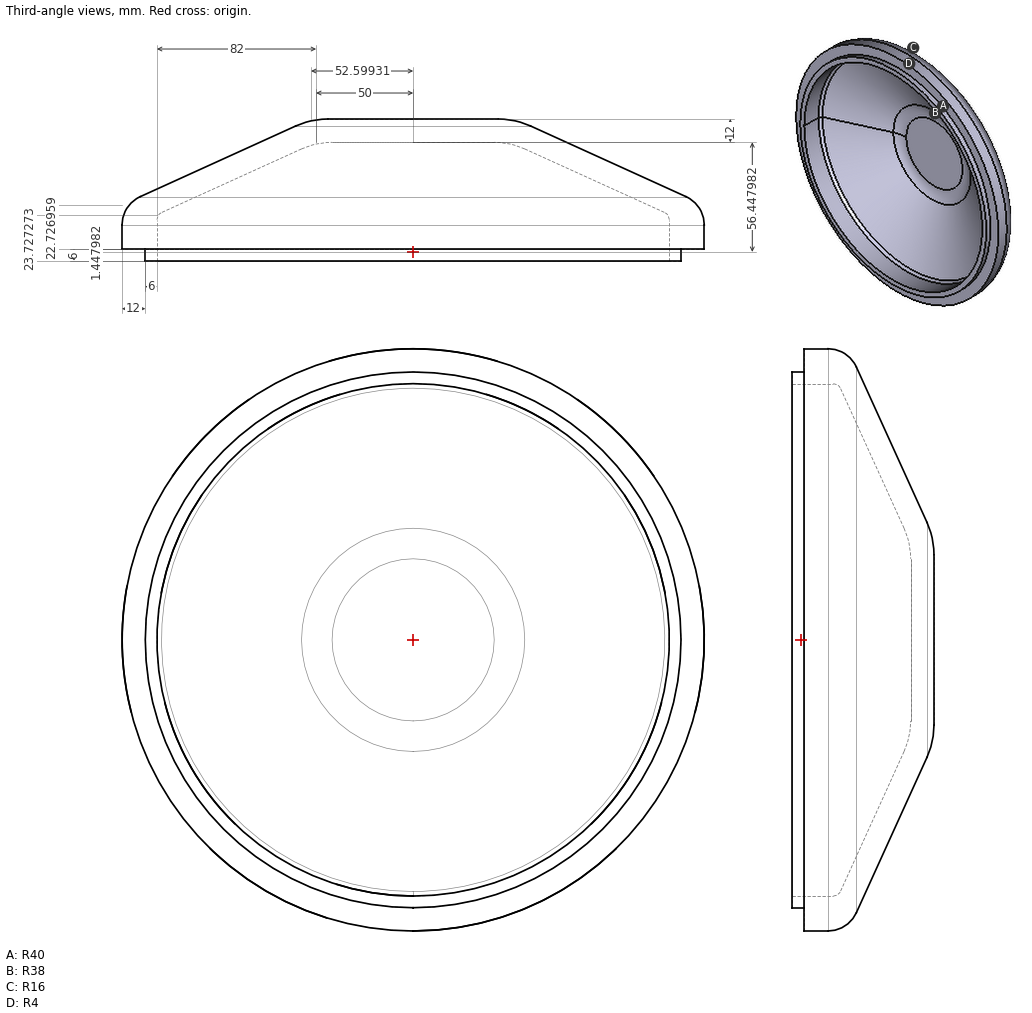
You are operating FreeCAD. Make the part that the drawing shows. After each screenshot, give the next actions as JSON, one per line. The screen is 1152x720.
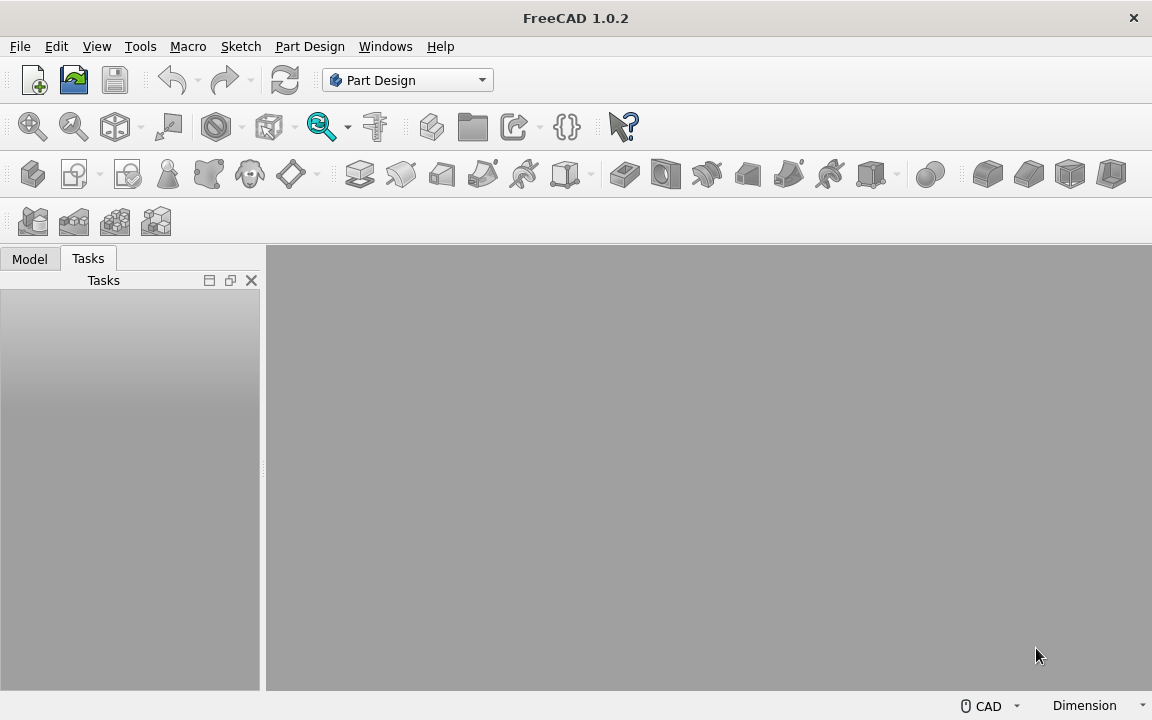
{"action": "key", "text": "ctrl+n"}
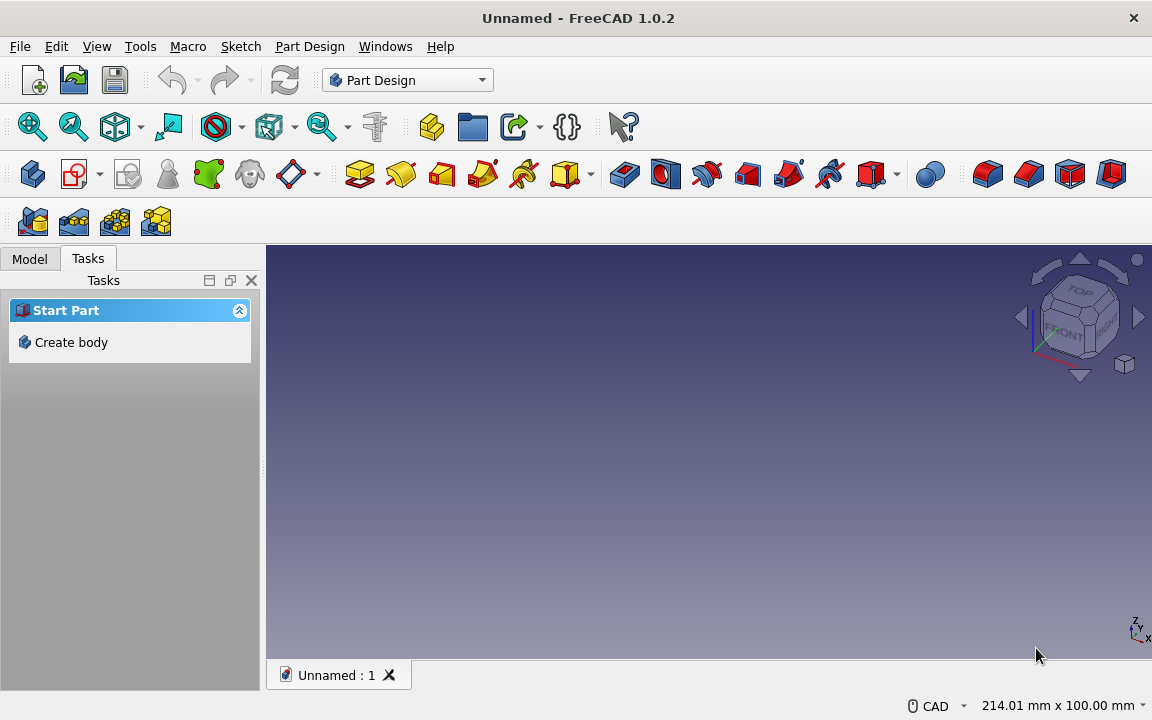
{"action": "left_click", "coordinate": [74, 174]}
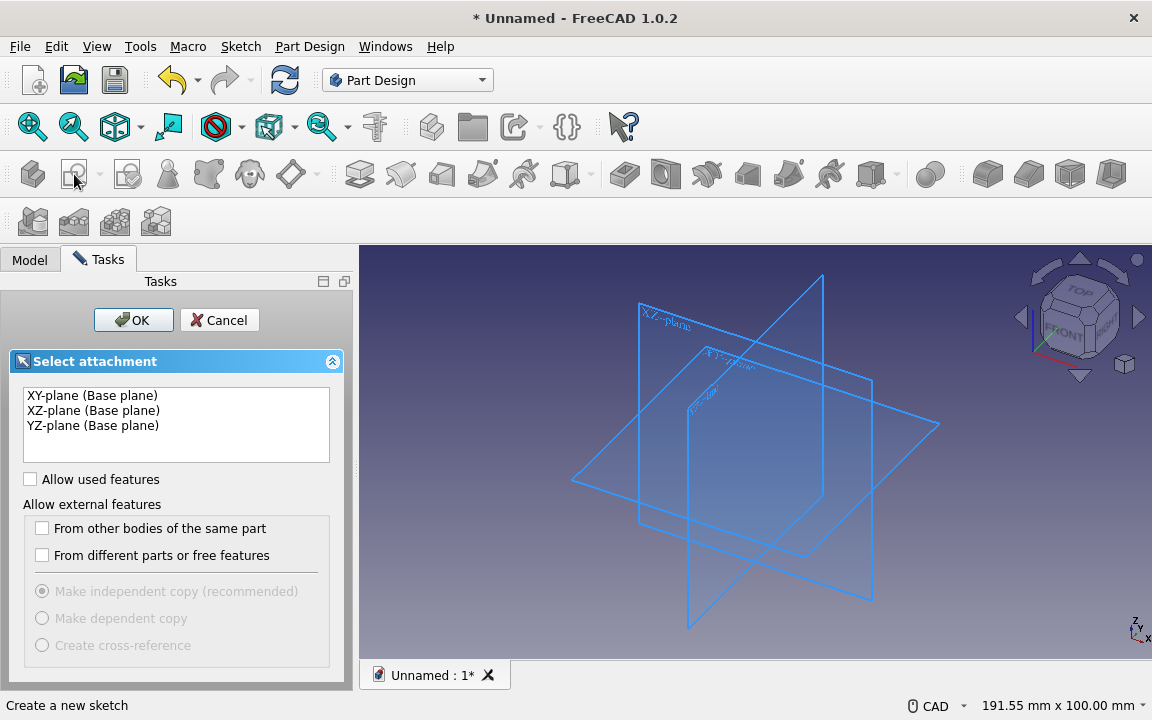
{"action": "left_click", "coordinate": [84, 396]}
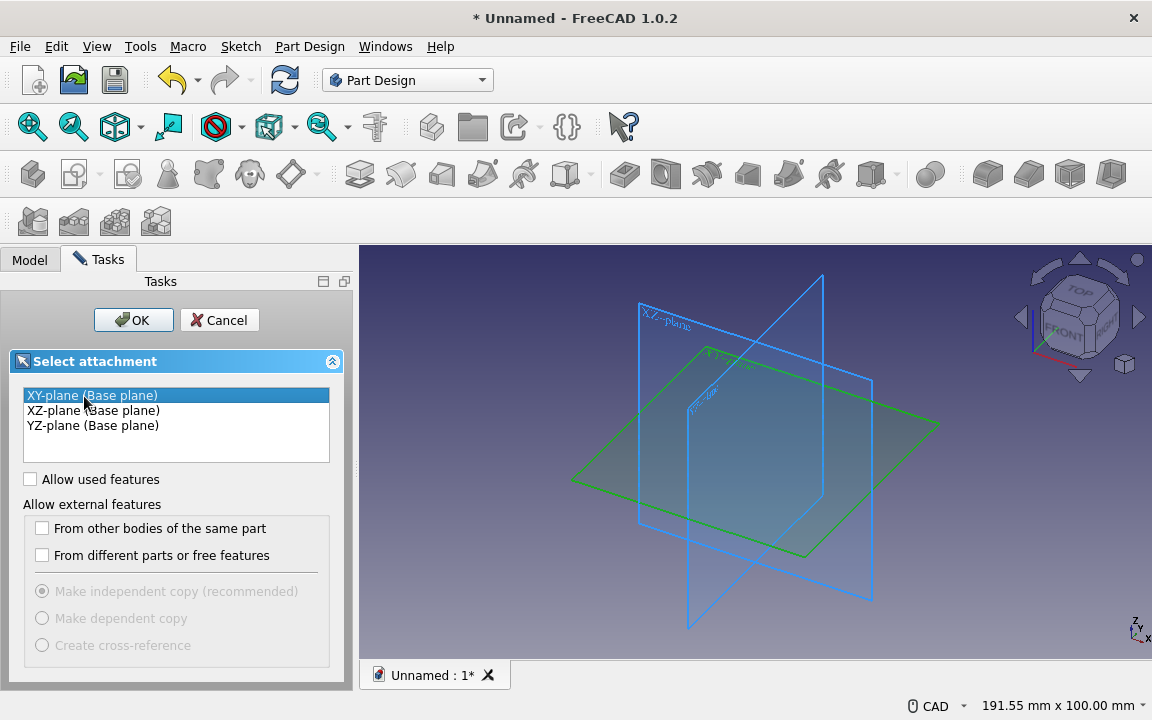
{"action": "left_click", "coordinate": [134, 320]}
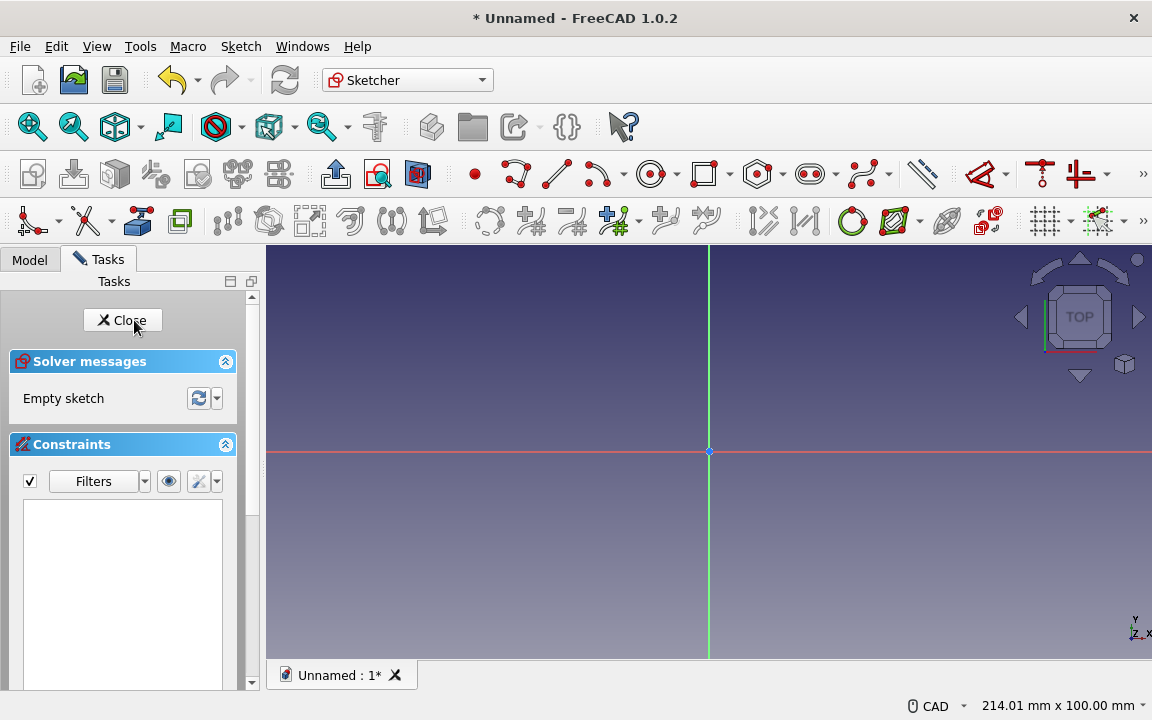
{"action": "scroll", "coordinate": [987, 631], "scroll_direction": "down", "scroll_amount": 2}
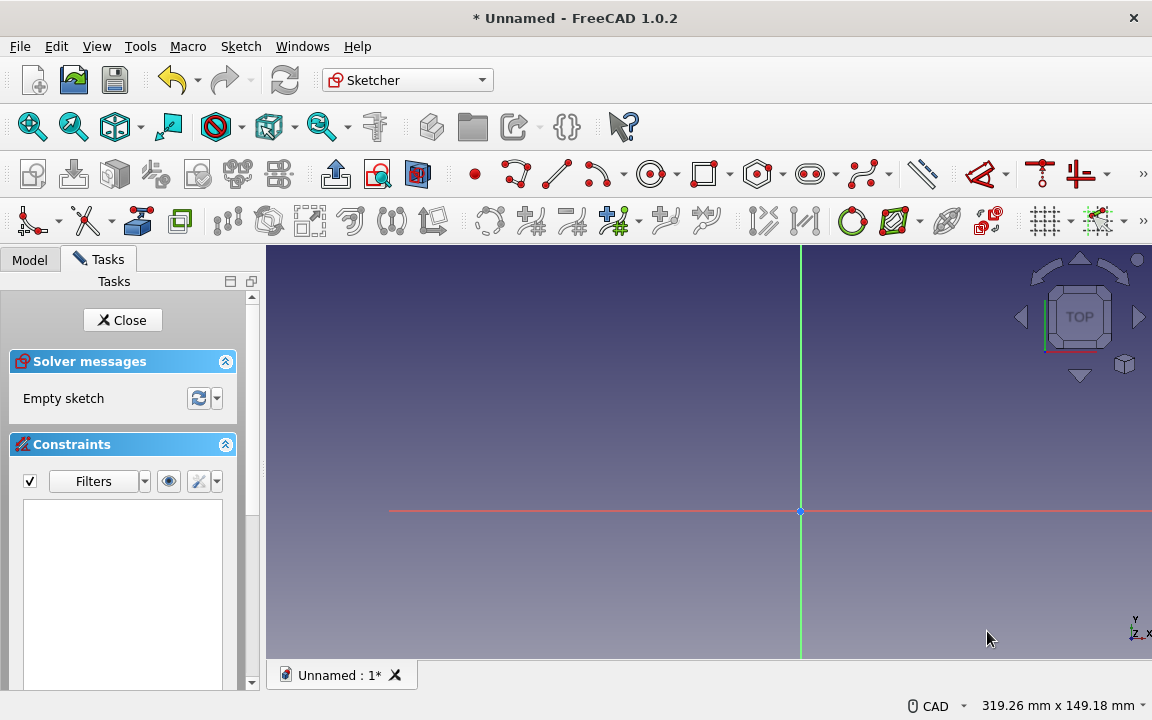
{"action": "key", "text": "g m"}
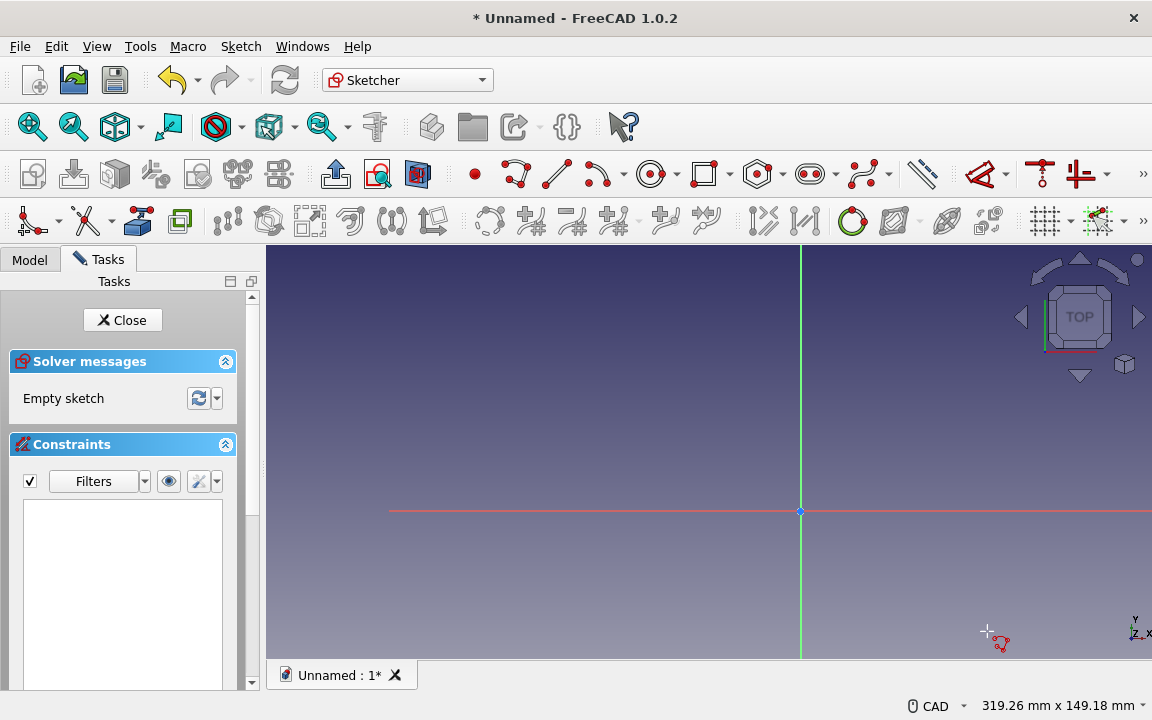
{"action": "left_click", "coordinate": [801, 355]}
{"action": "left_click", "coordinate": [792, 321]}
{"action": "left_click", "coordinate": [655, 321]}
{"action": "left_click", "coordinate": [385, 444]}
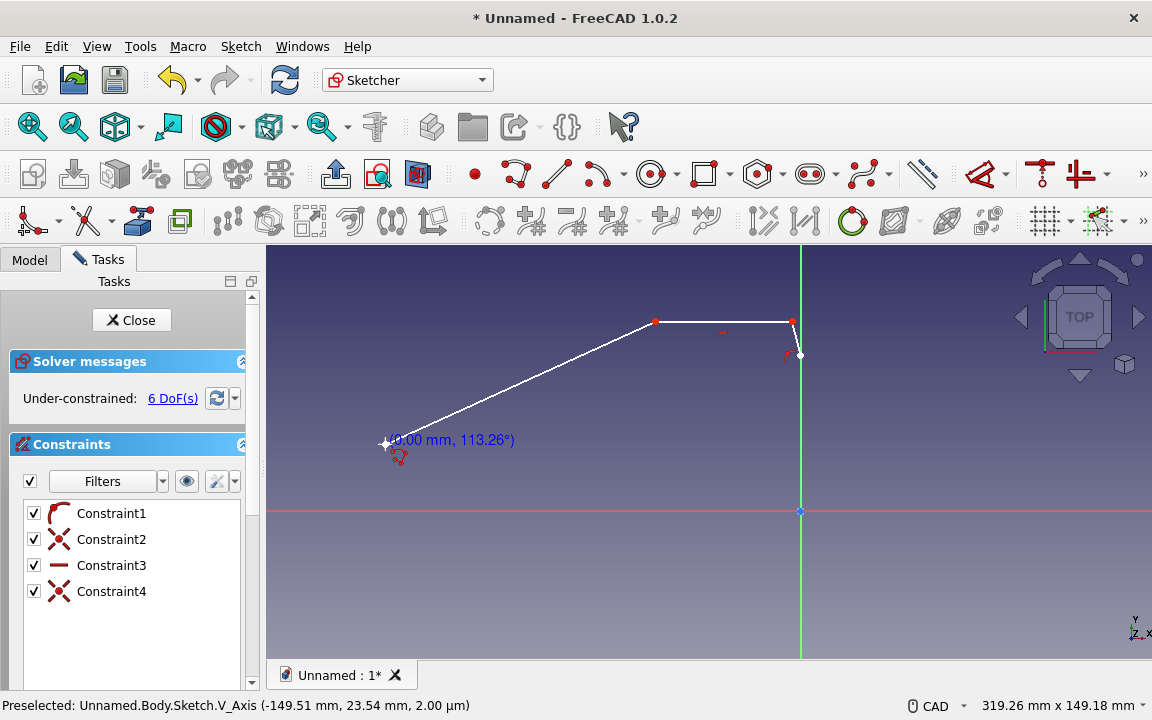
{"action": "scroll", "coordinate": [385, 507], "scroll_direction": "up", "scroll_amount": 7}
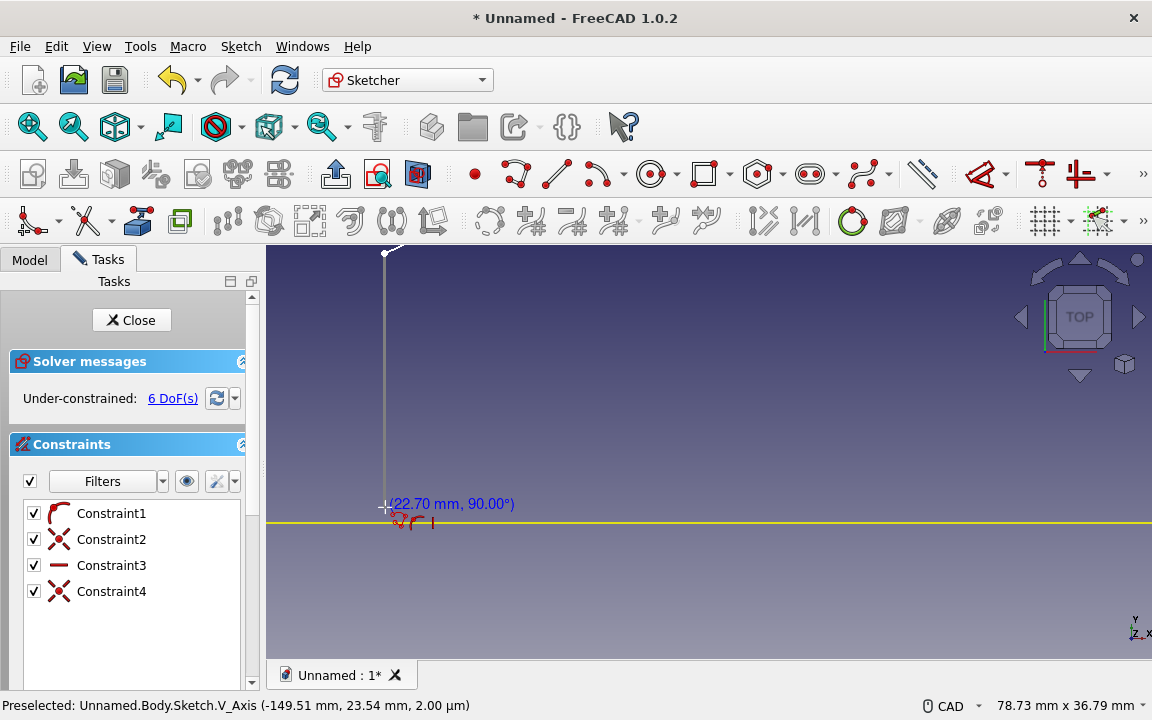
{"action": "left_click", "coordinate": [385, 506]}
{"action": "left_click", "coordinate": [518, 506]}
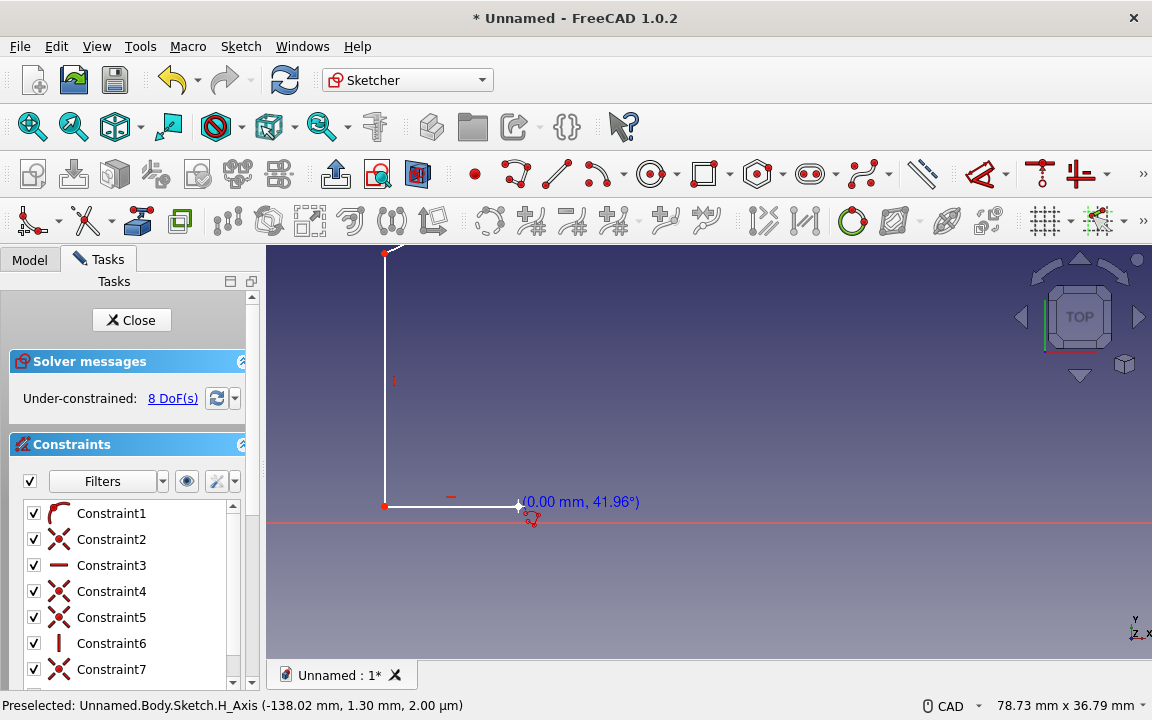
{"action": "scroll", "coordinate": [388, 577], "scroll_direction": "down", "scroll_amount": 6}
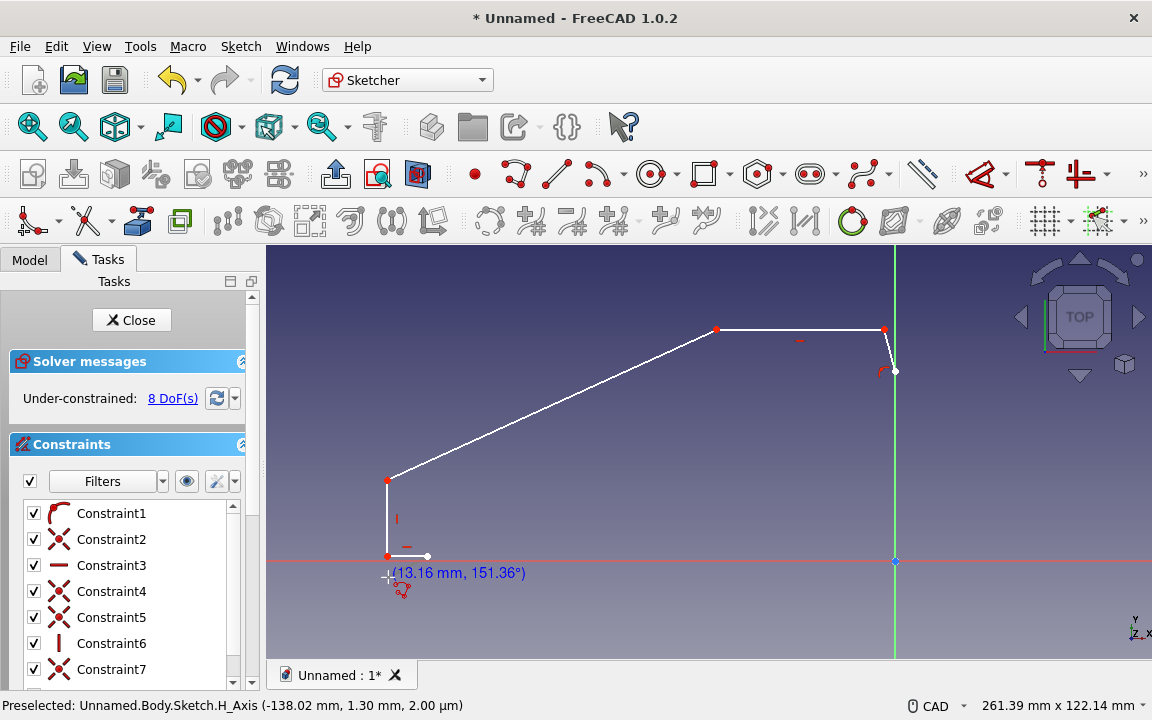
{"action": "left_click", "coordinate": [427, 577]}
{"action": "left_click", "coordinate": [448, 577]}
{"action": "left_click", "coordinate": [448, 496]}
{"action": "left_click", "coordinate": [726, 370]}
{"action": "left_click", "coordinate": [895, 371]}
{"action": "key", "text": "Escape"}
{"action": "key", "text": "Escape"}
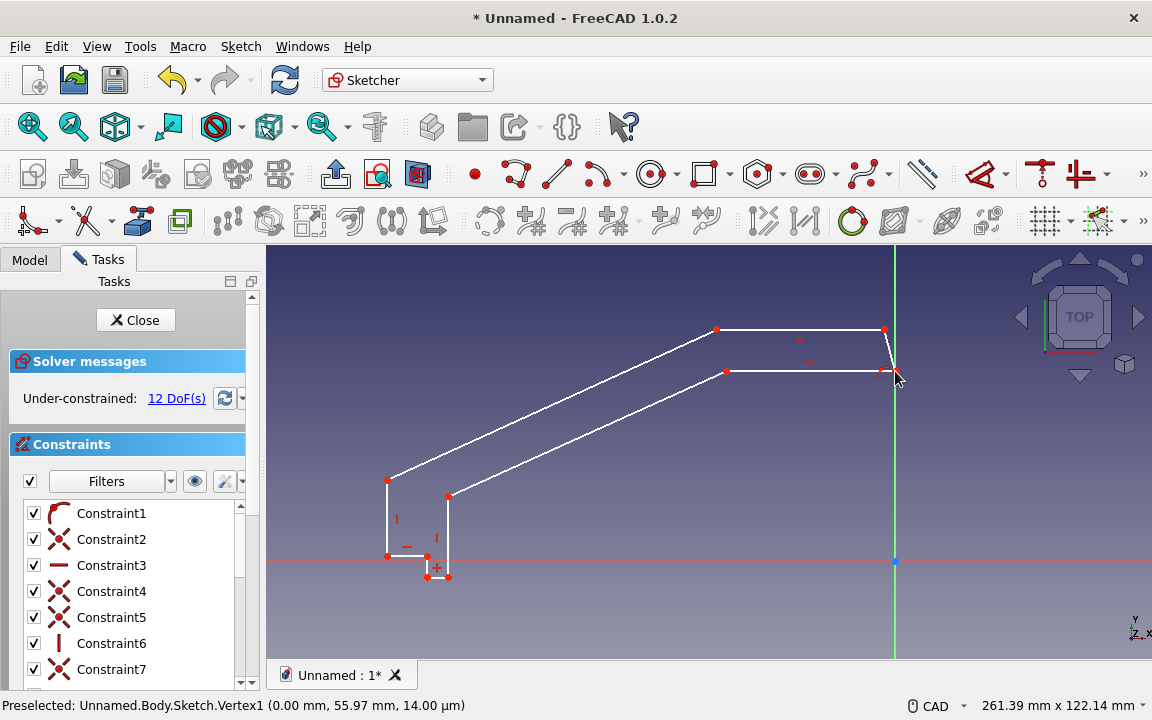
{"action": "left_click", "coordinate": [892, 359]}